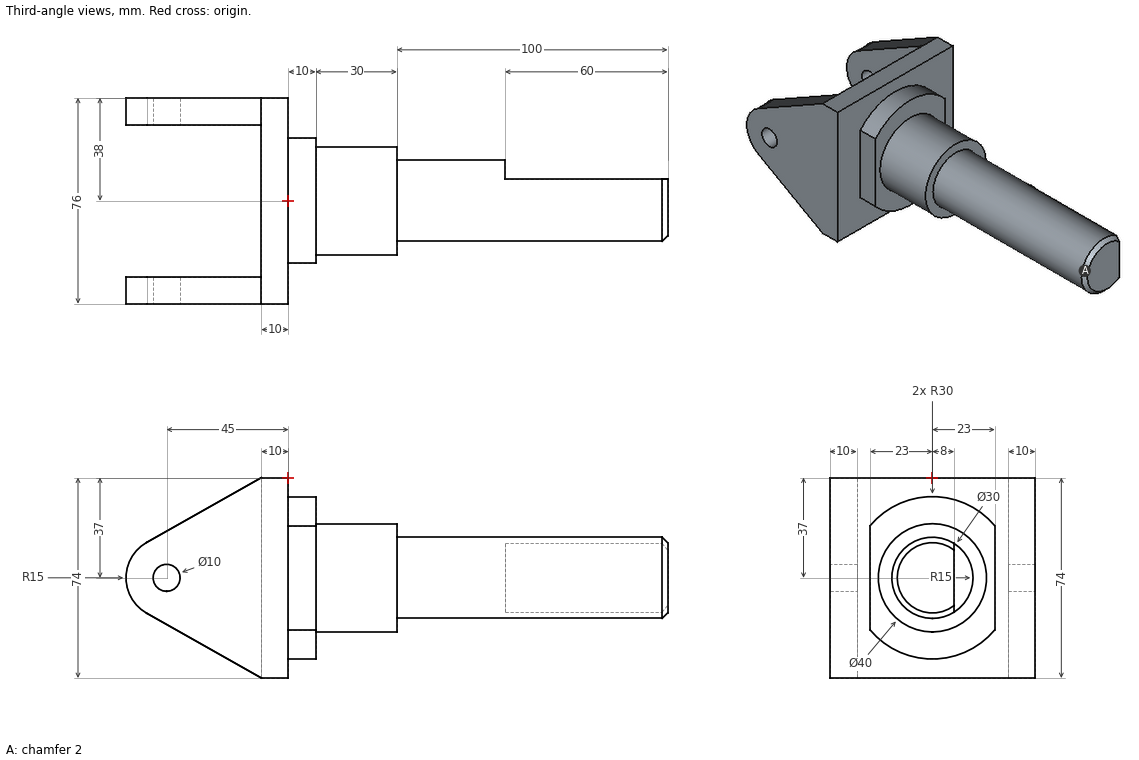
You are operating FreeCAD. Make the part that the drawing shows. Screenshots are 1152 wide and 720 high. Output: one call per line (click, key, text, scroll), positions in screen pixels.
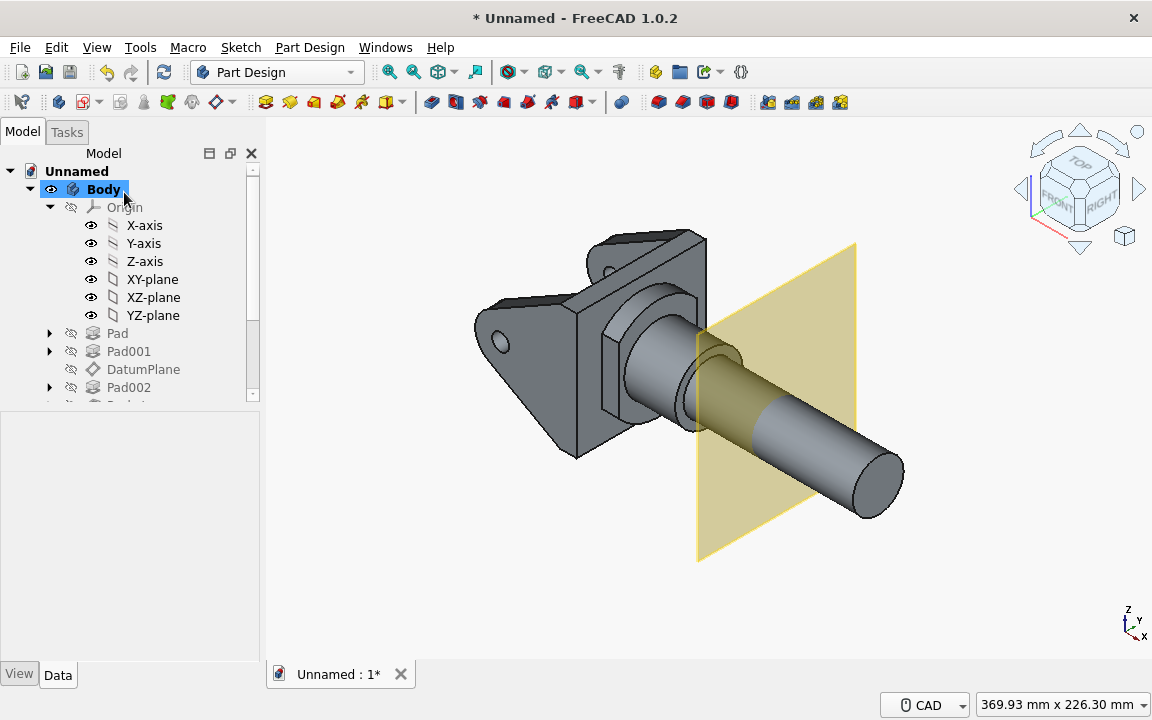
scroll(100, 275, down, 3)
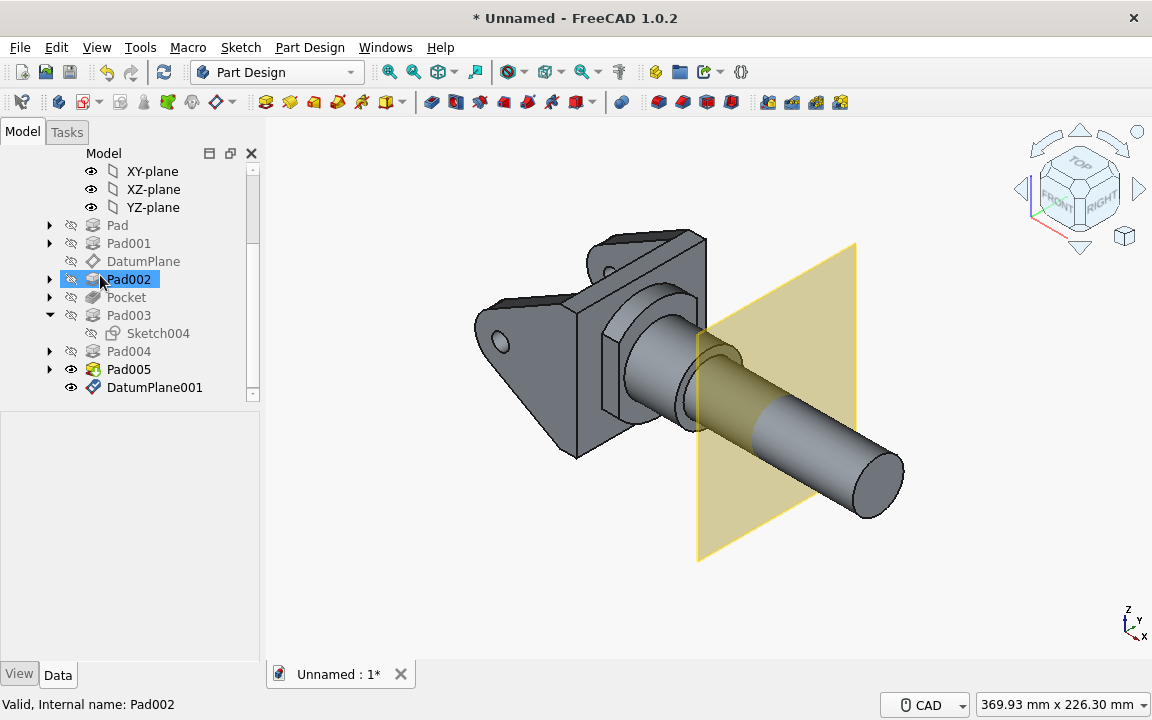
click(116, 387)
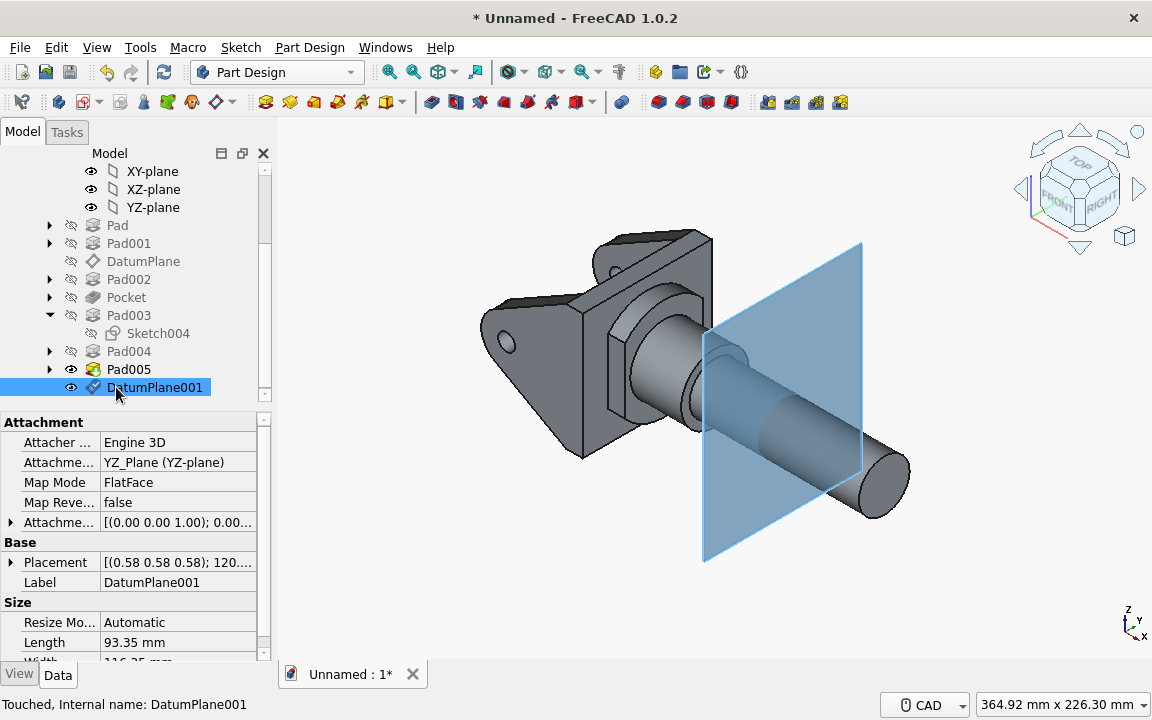
click(84, 102)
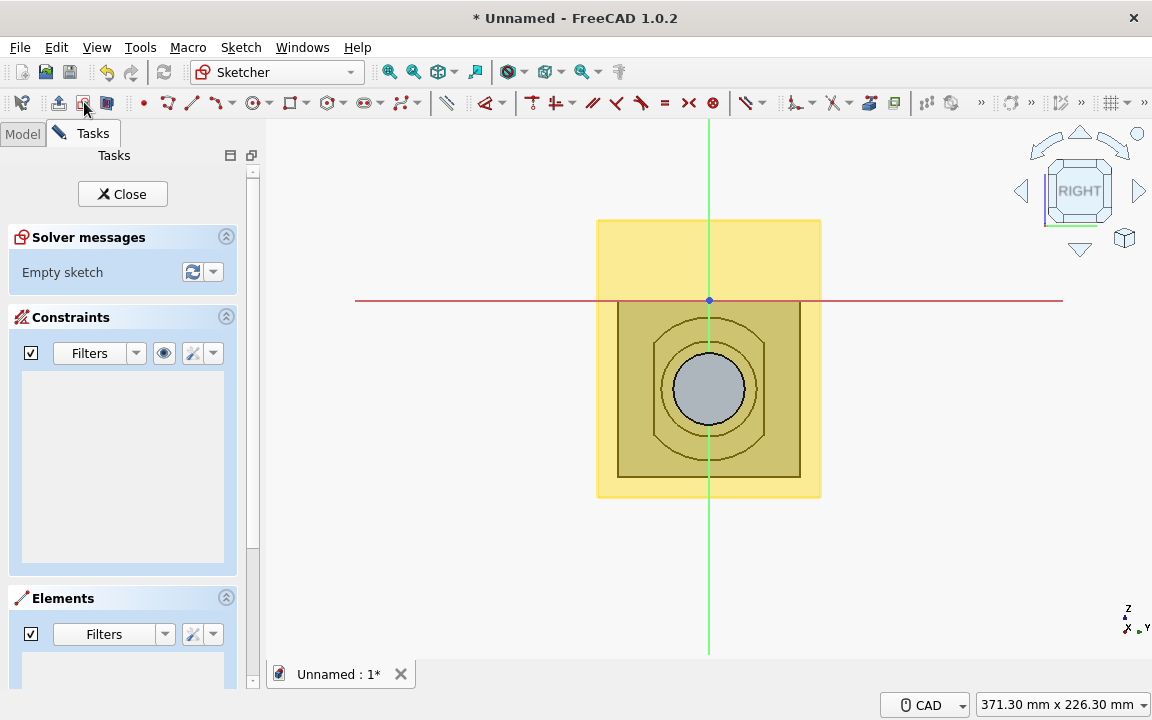
key(q)
key(s)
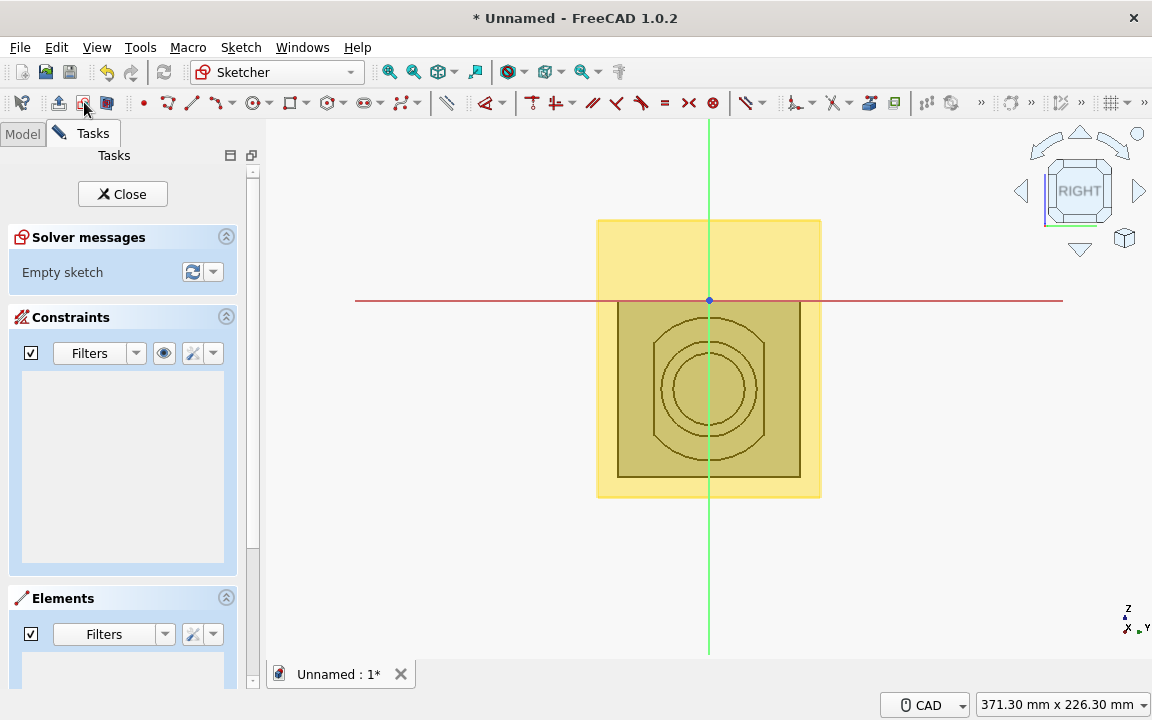
scroll(777, 343, up, 5)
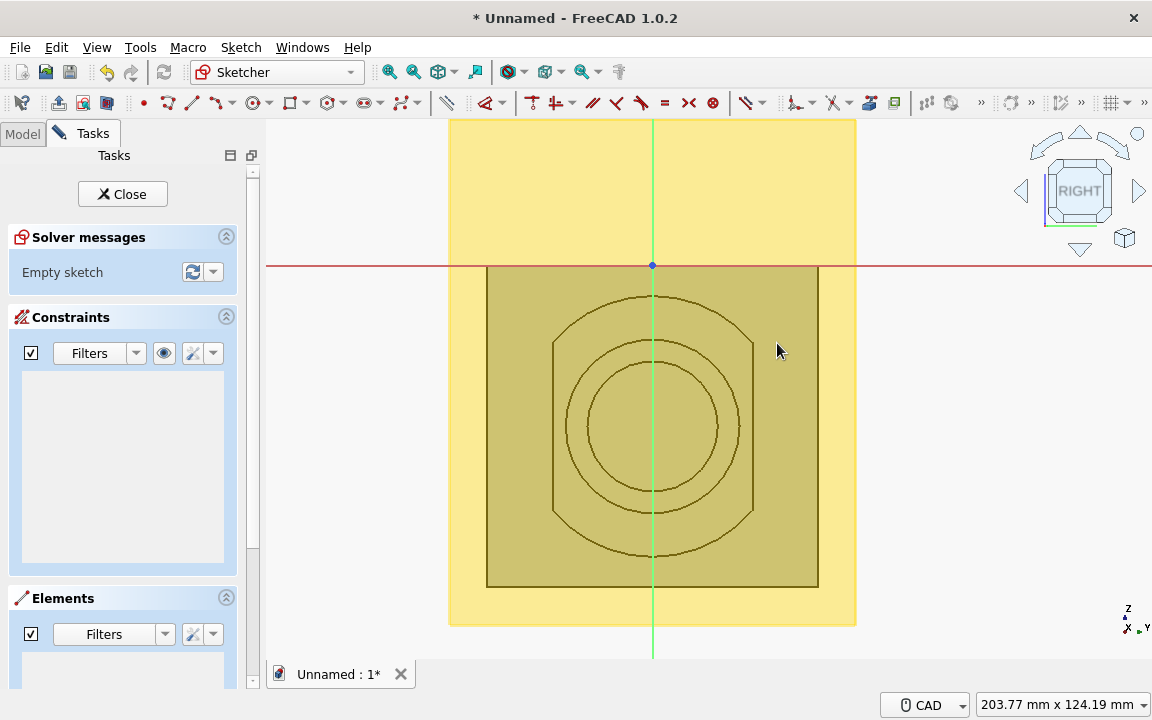
click(192, 104)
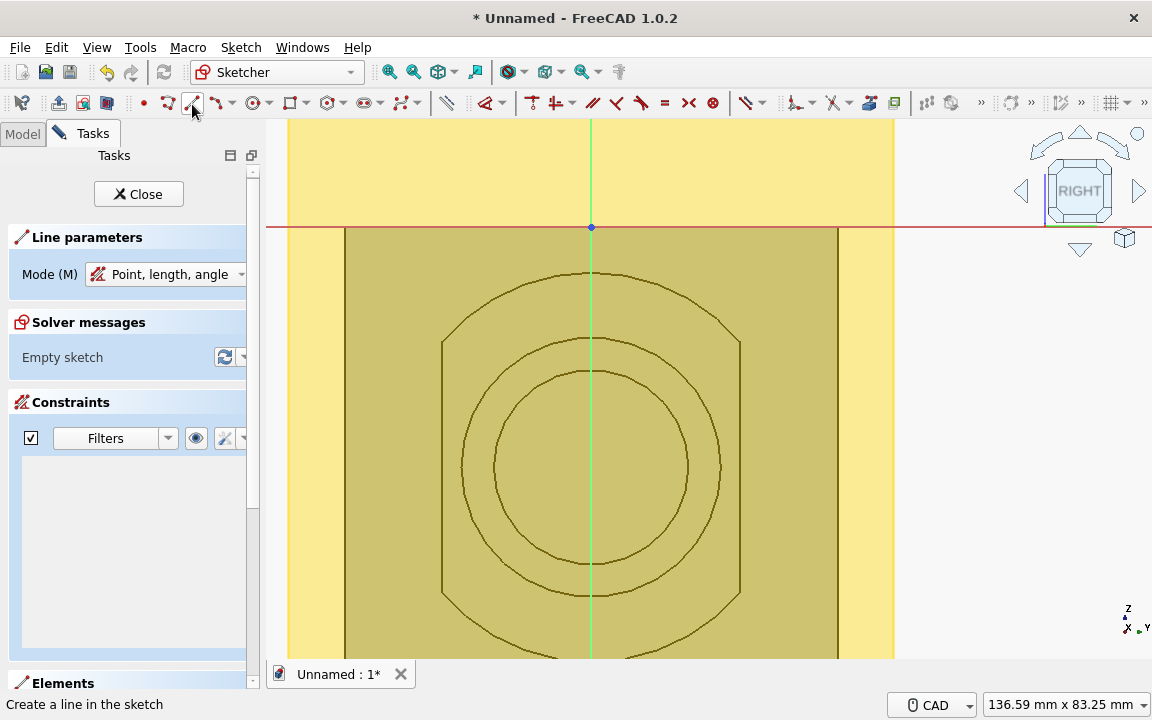
click(643, 385)
click(643, 550)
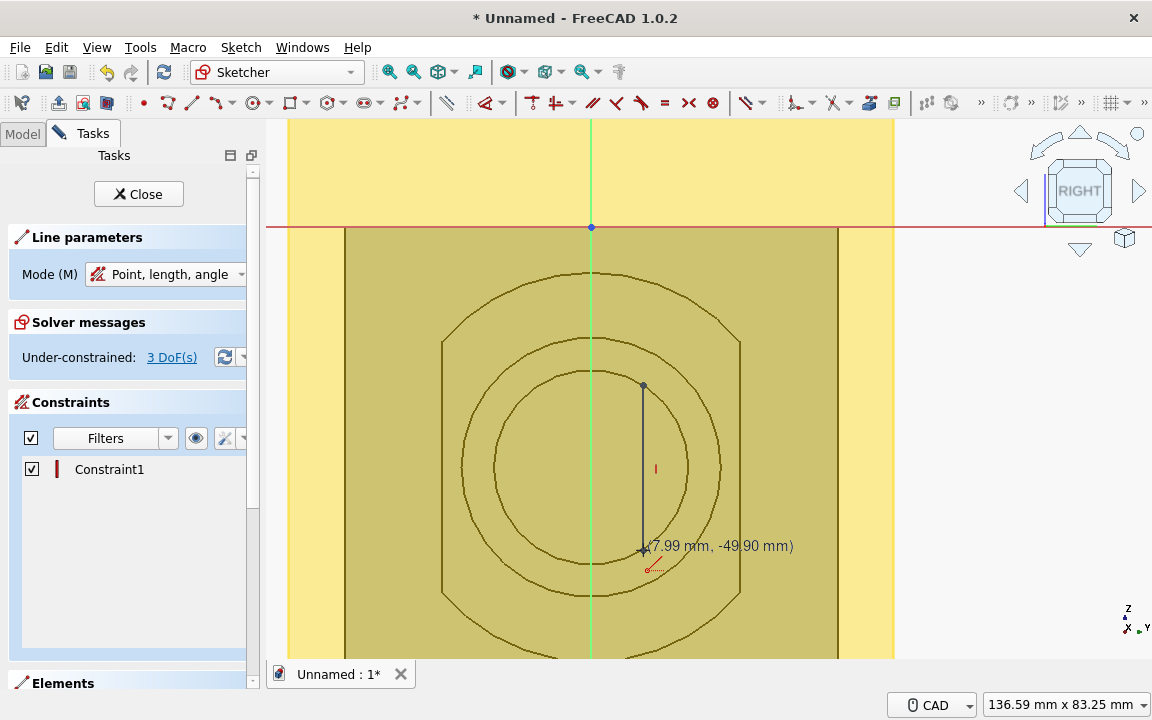
click(216, 104)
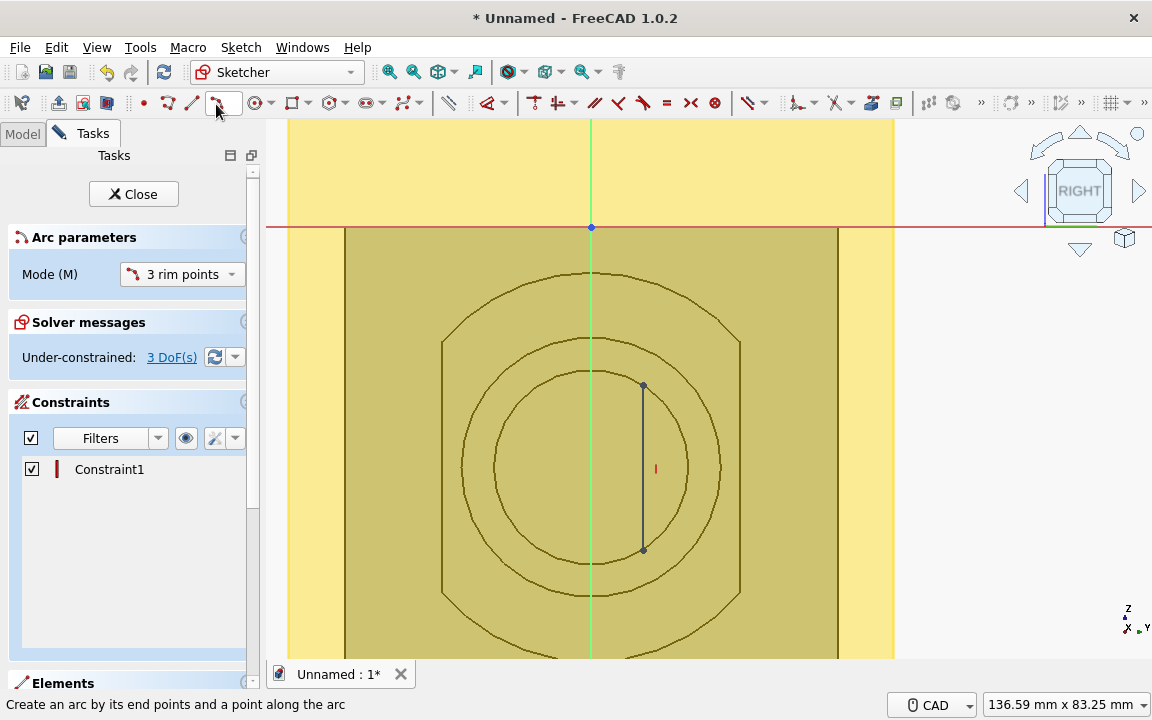
click(643, 551)
click(643, 386)
click(688, 467)
key(Escape)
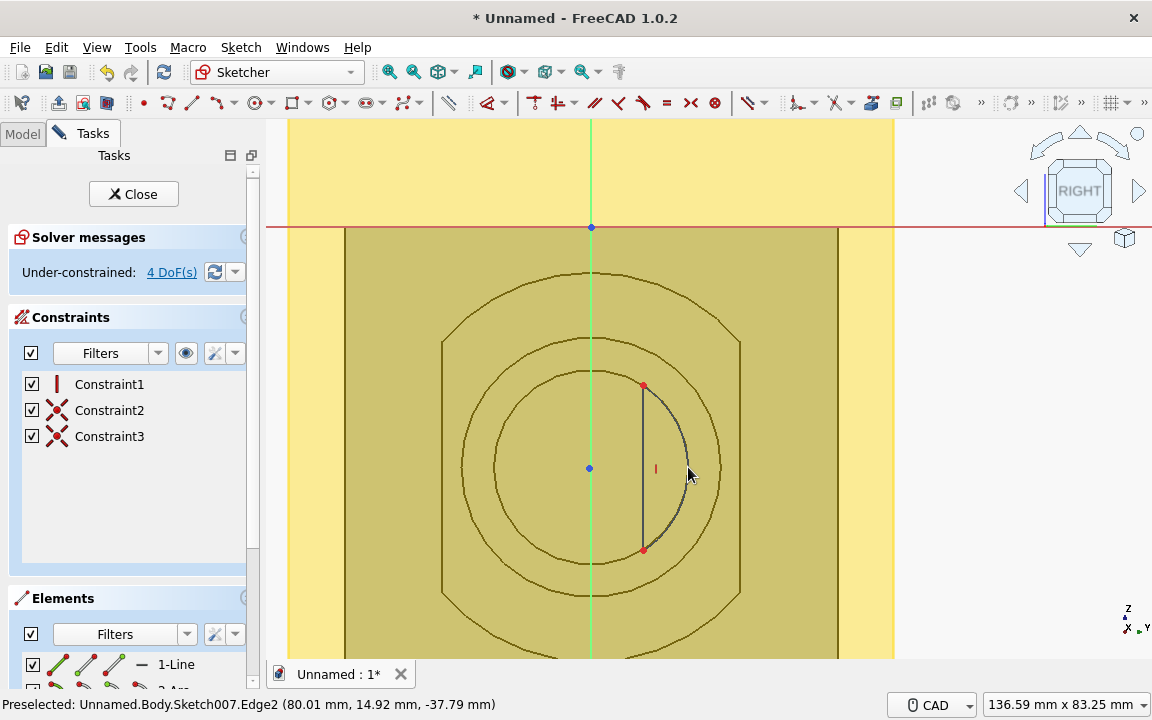
click(590, 468)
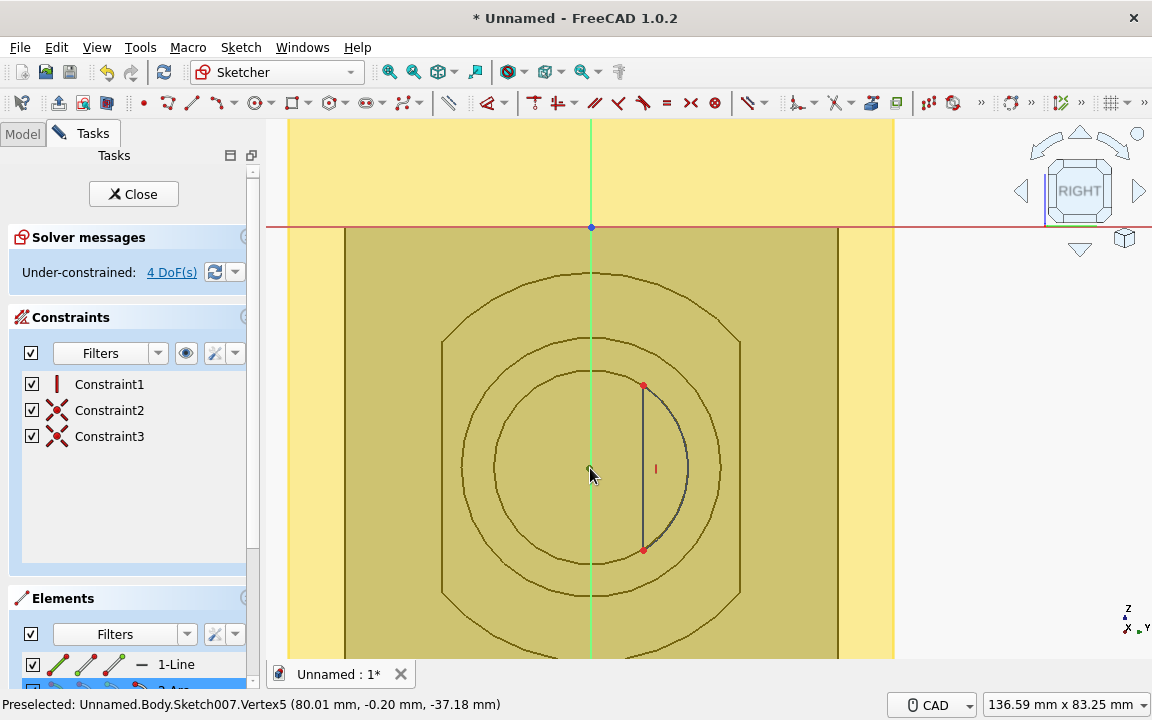
click(591, 596)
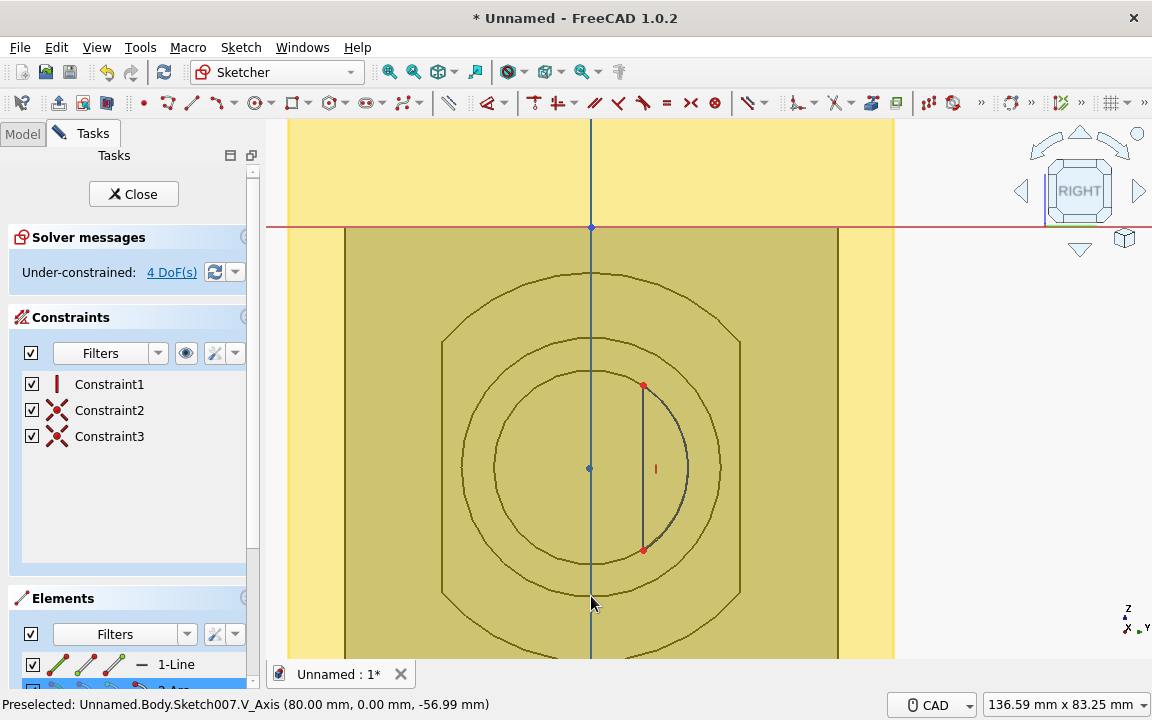
click(534, 104)